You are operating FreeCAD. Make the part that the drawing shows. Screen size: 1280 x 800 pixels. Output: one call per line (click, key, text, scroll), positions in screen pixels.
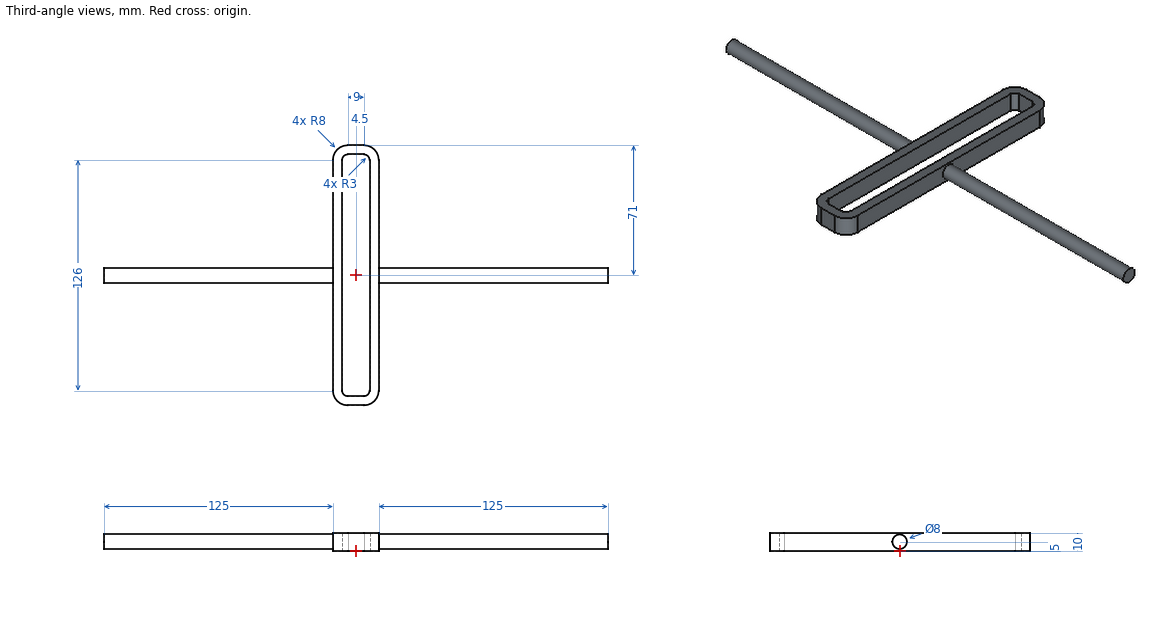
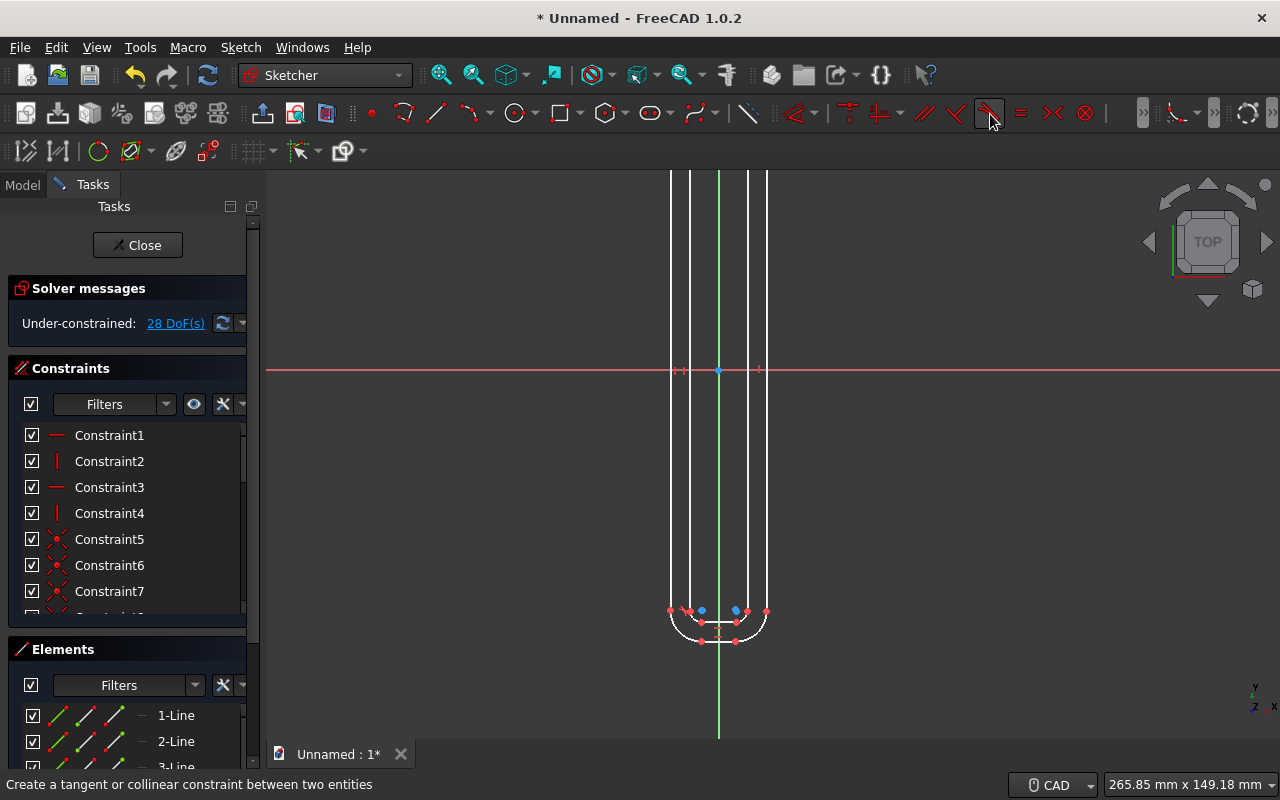
click(715, 642)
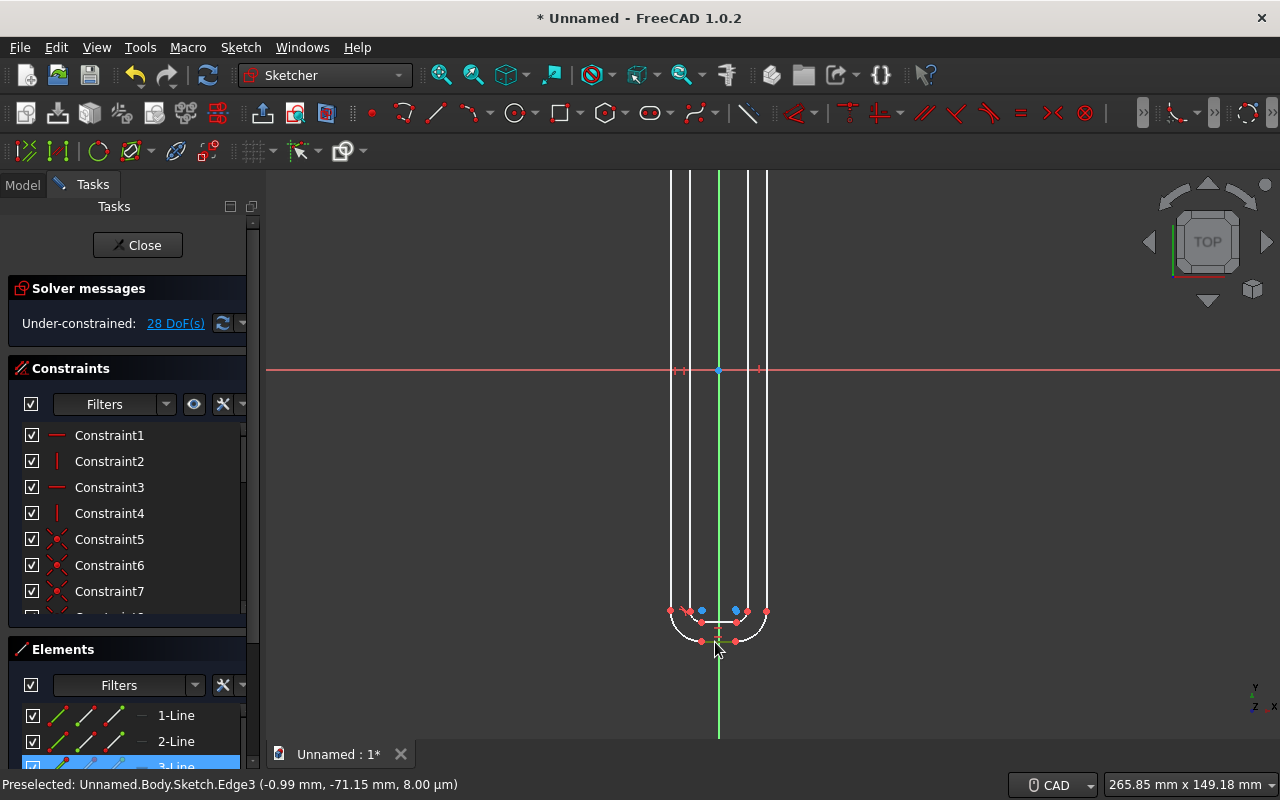
click(674, 625)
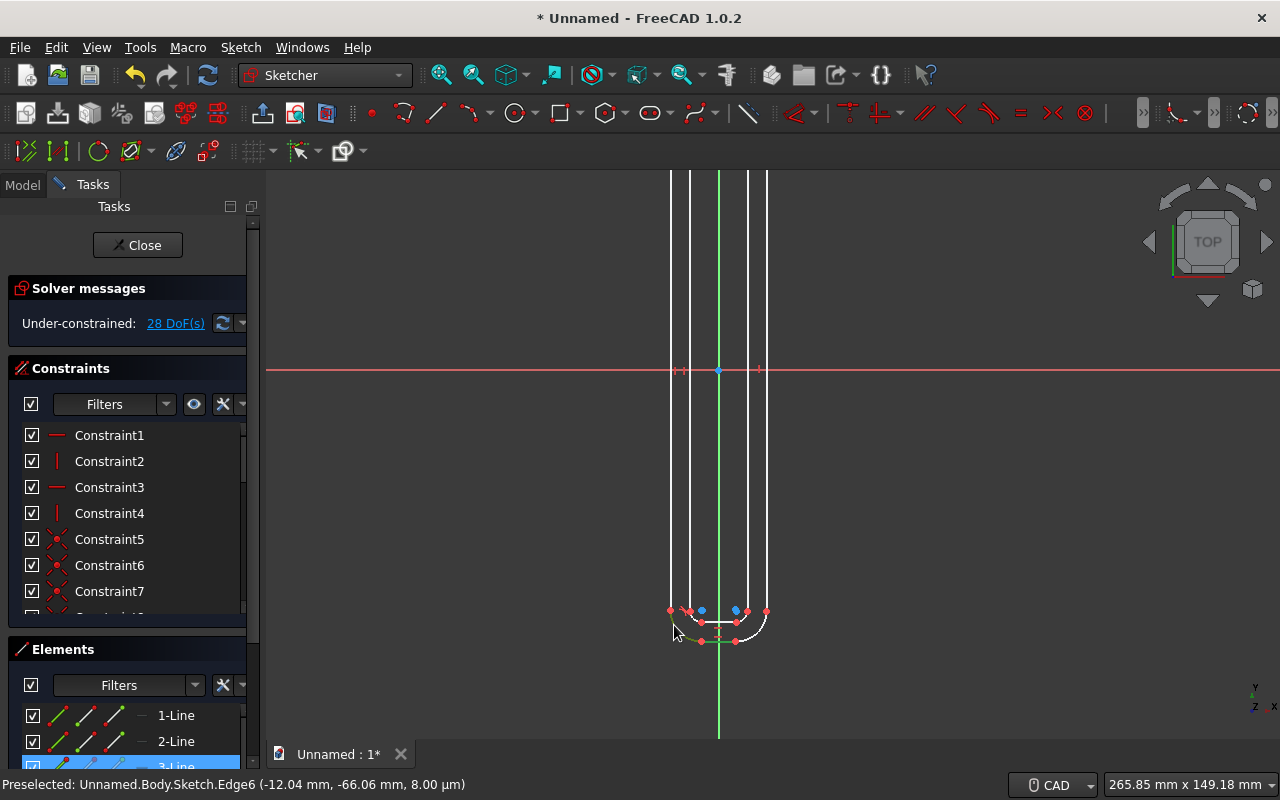
click(990, 114)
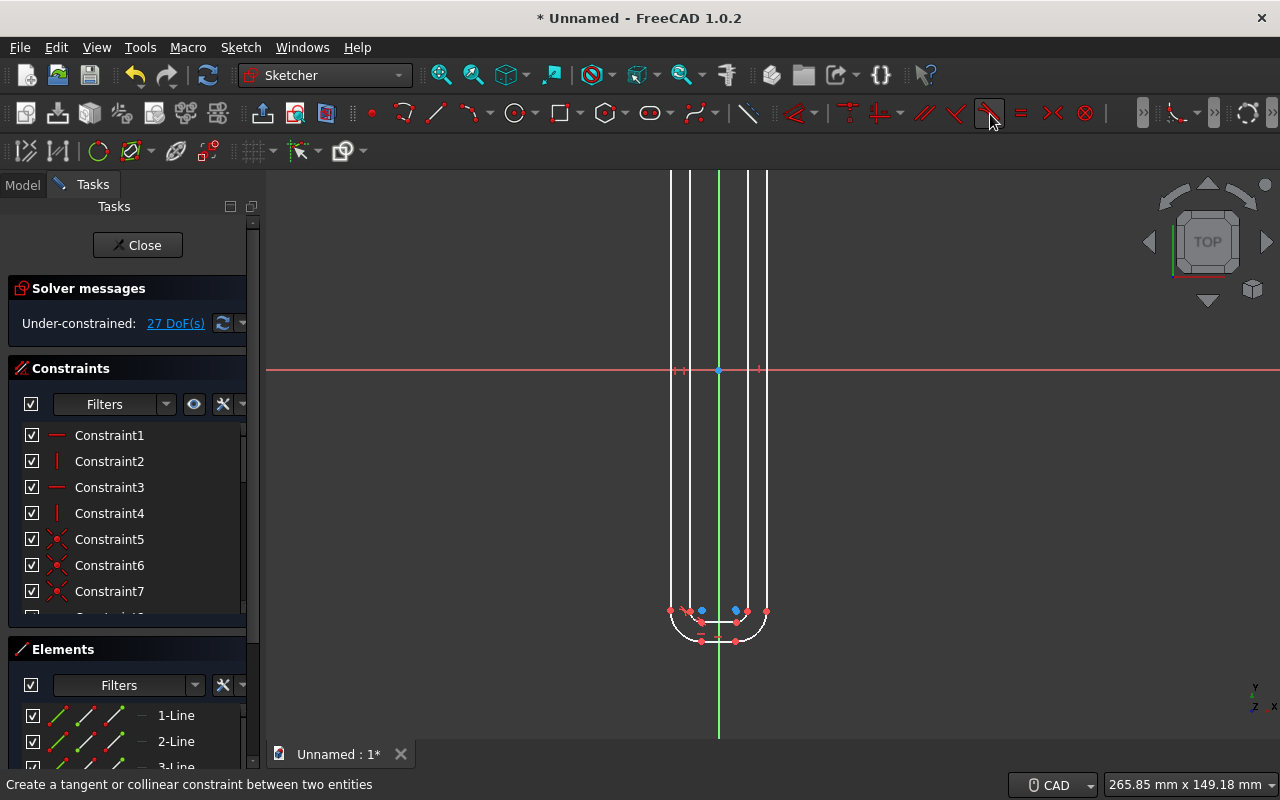
click(715, 642)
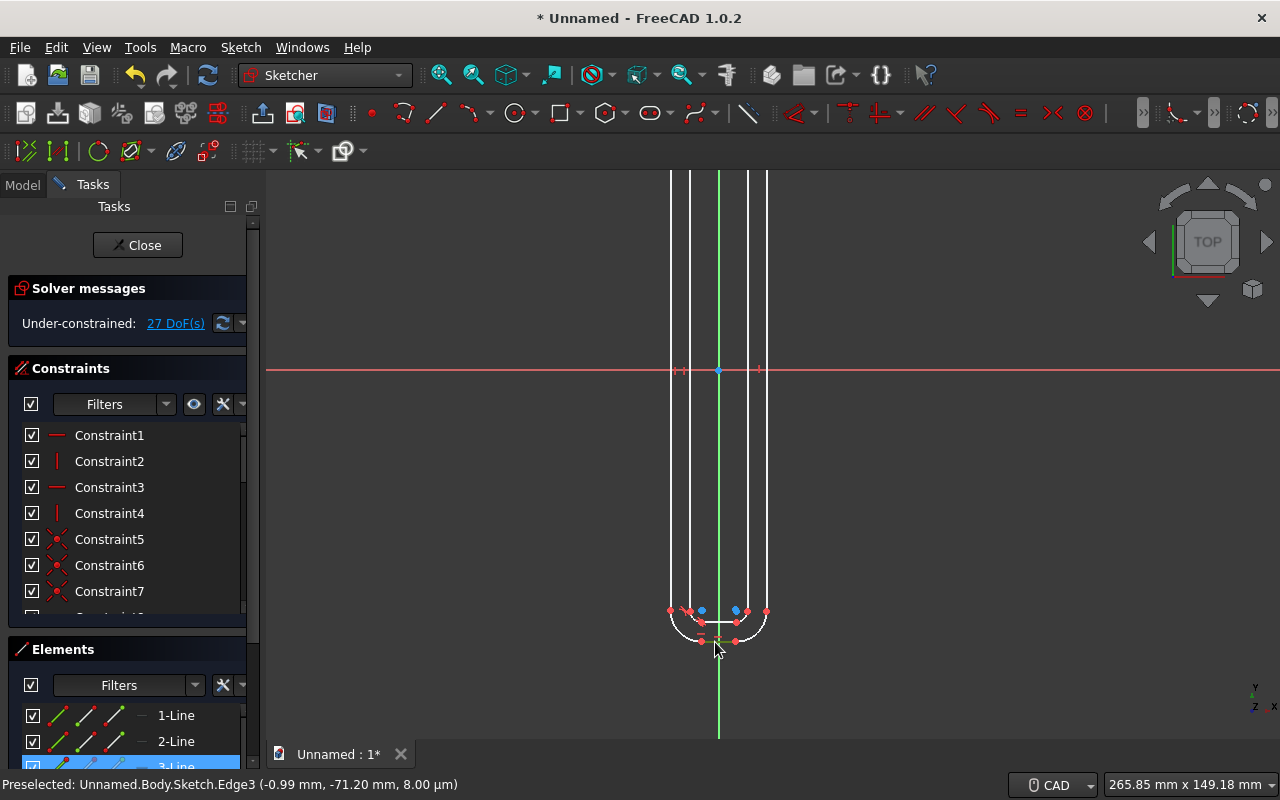
click(750, 639)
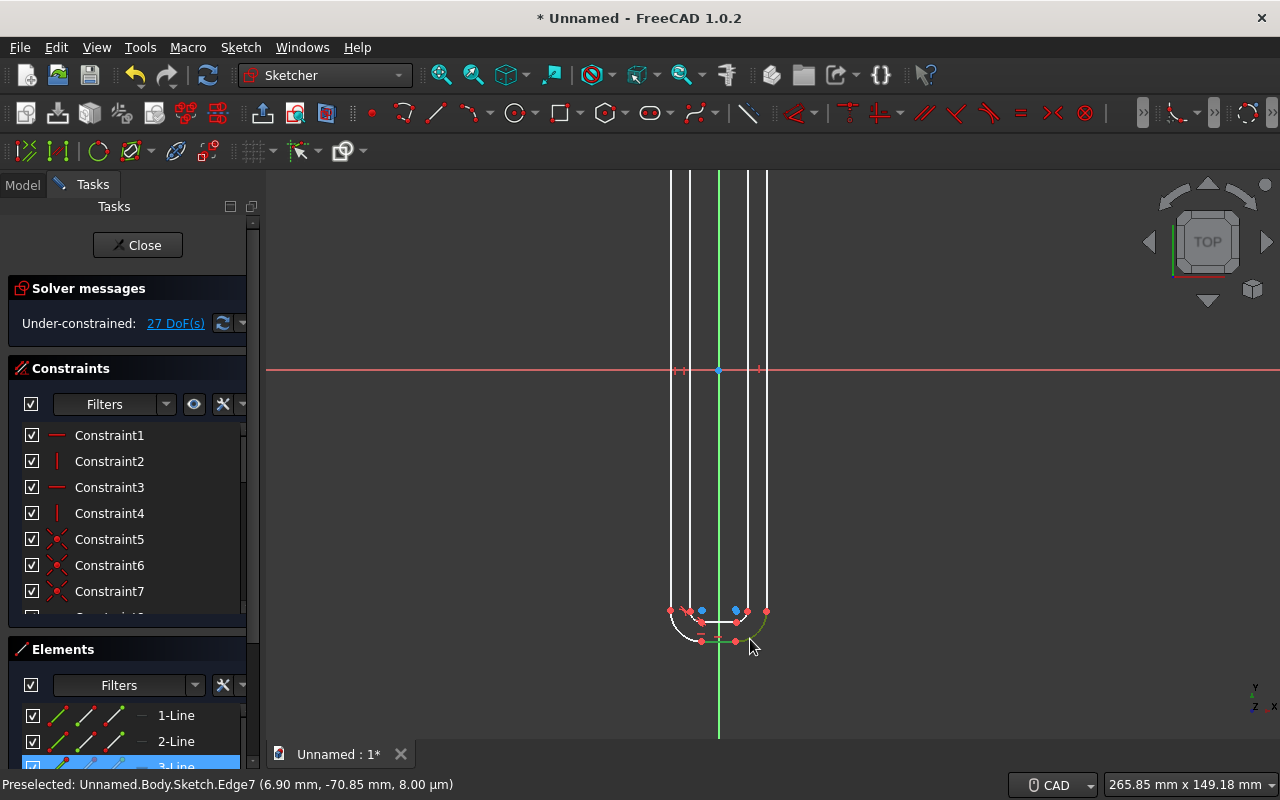
click(990, 114)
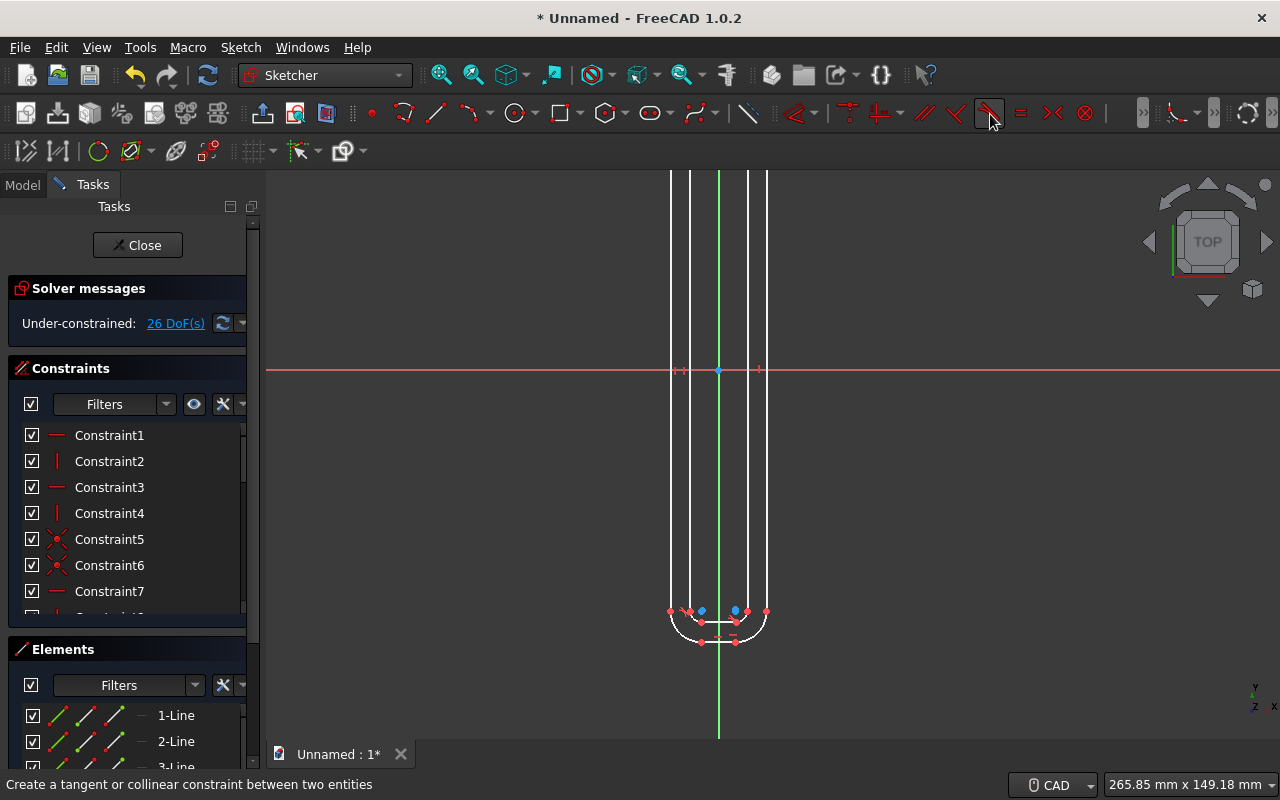
click(767, 467)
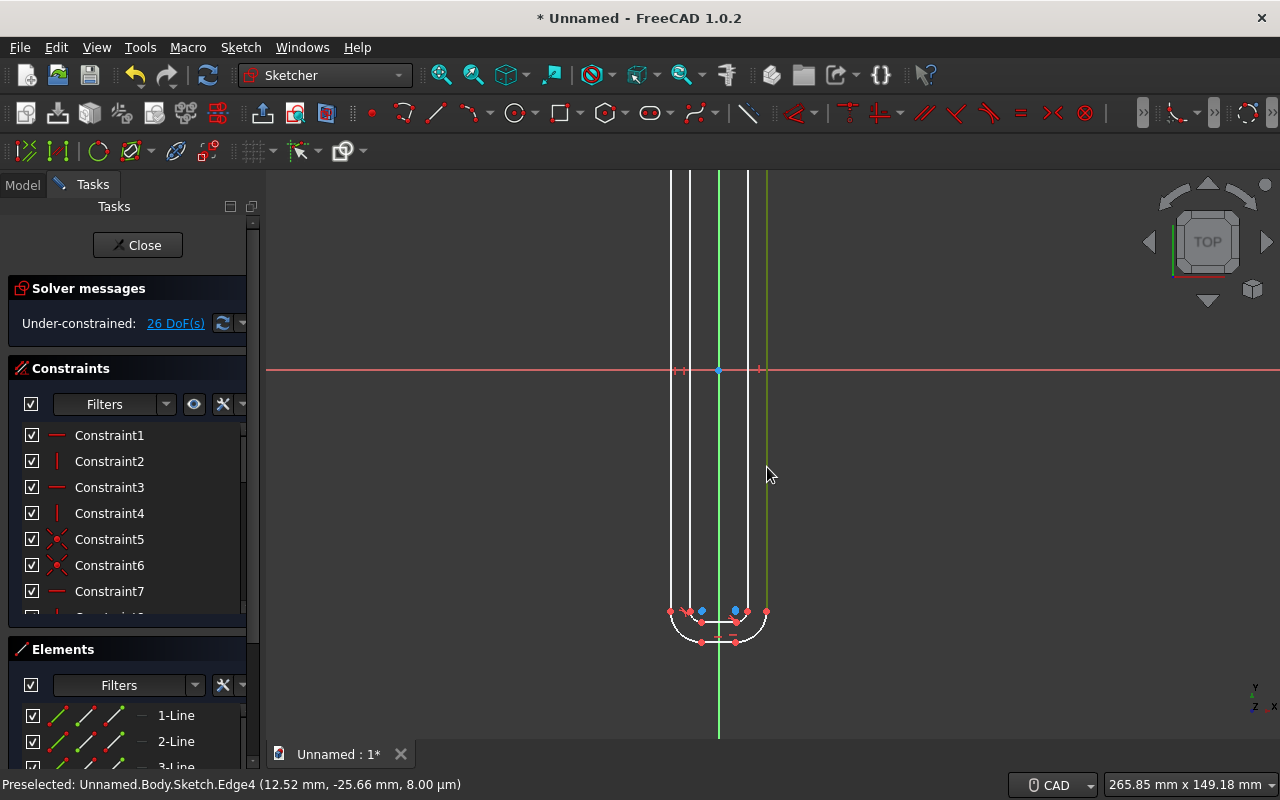
click(750, 639)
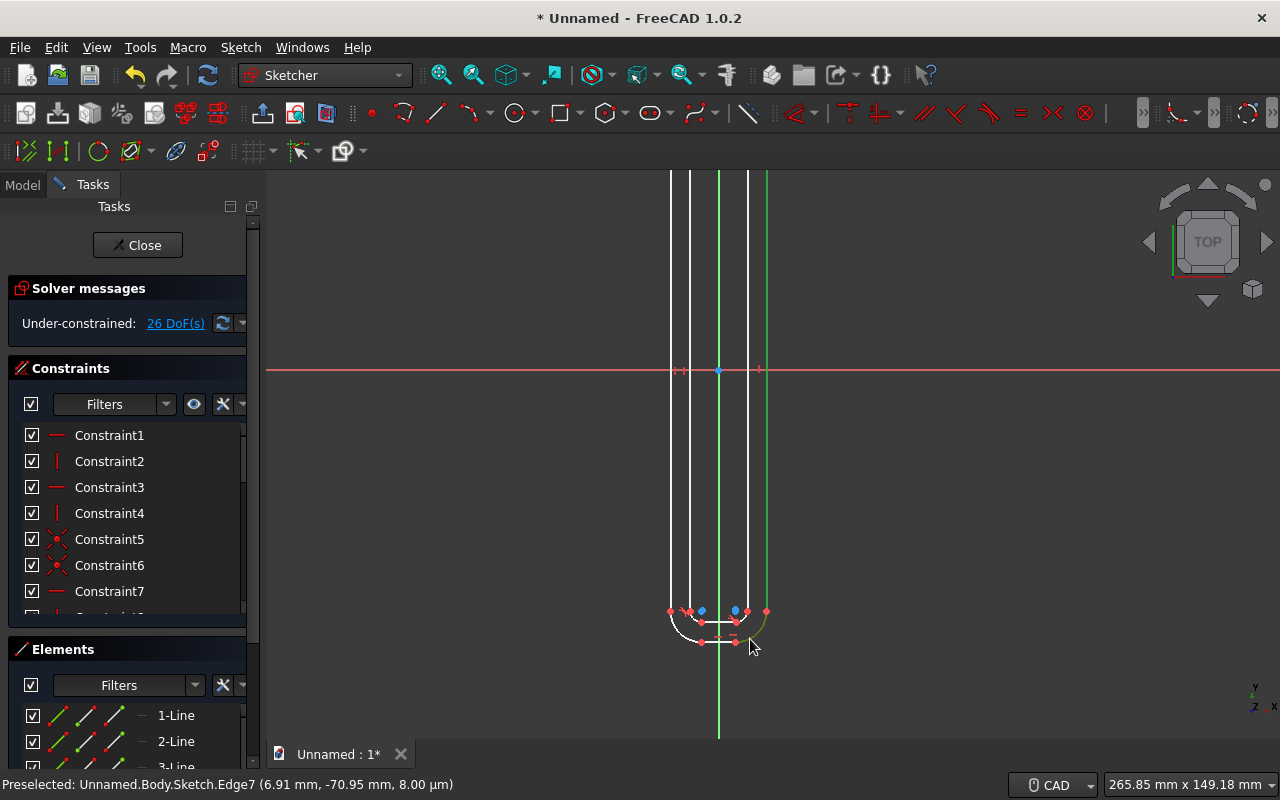
click(990, 114)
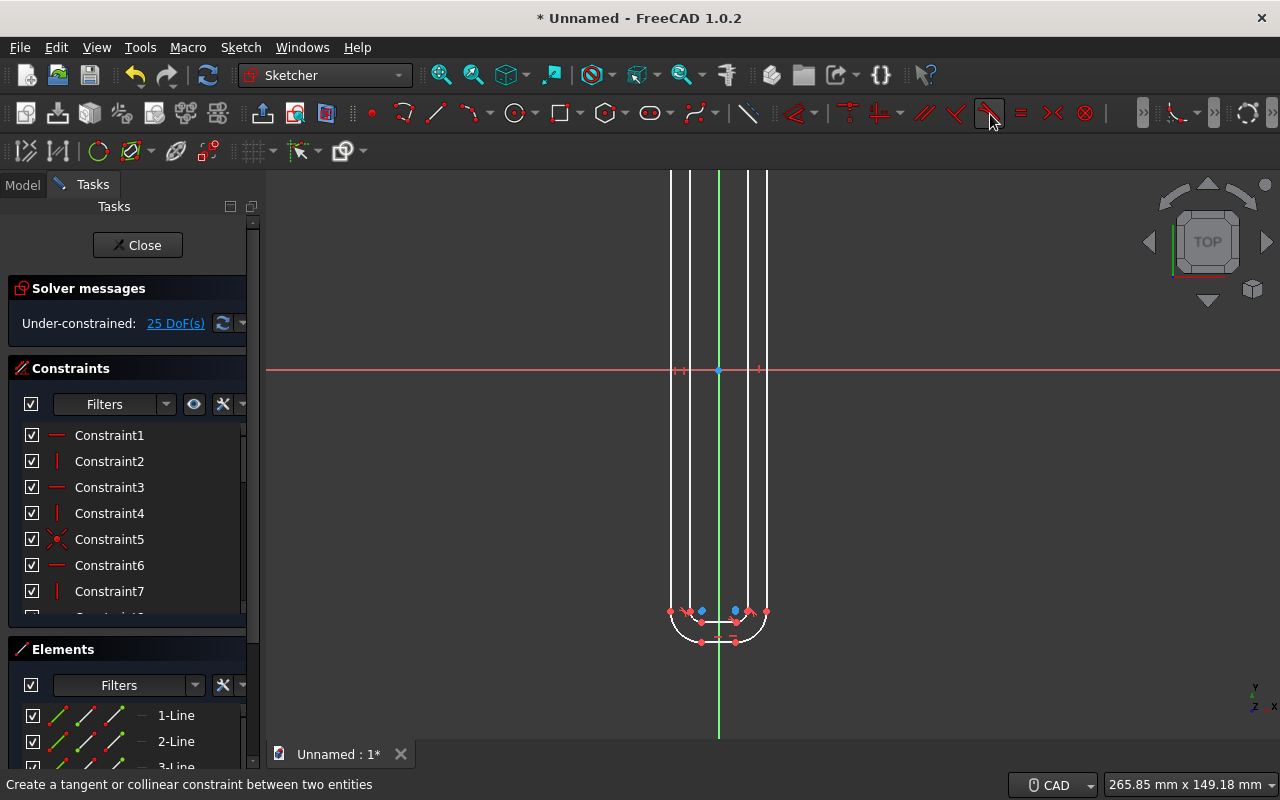
click(767, 467)